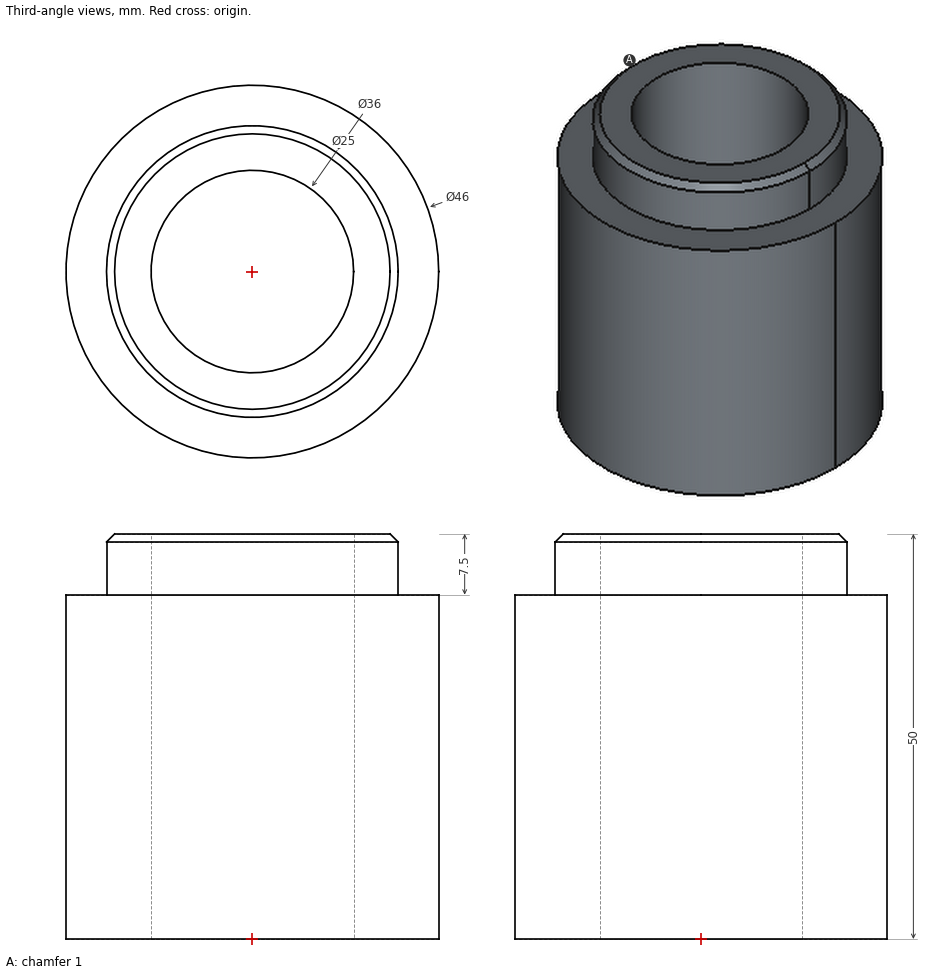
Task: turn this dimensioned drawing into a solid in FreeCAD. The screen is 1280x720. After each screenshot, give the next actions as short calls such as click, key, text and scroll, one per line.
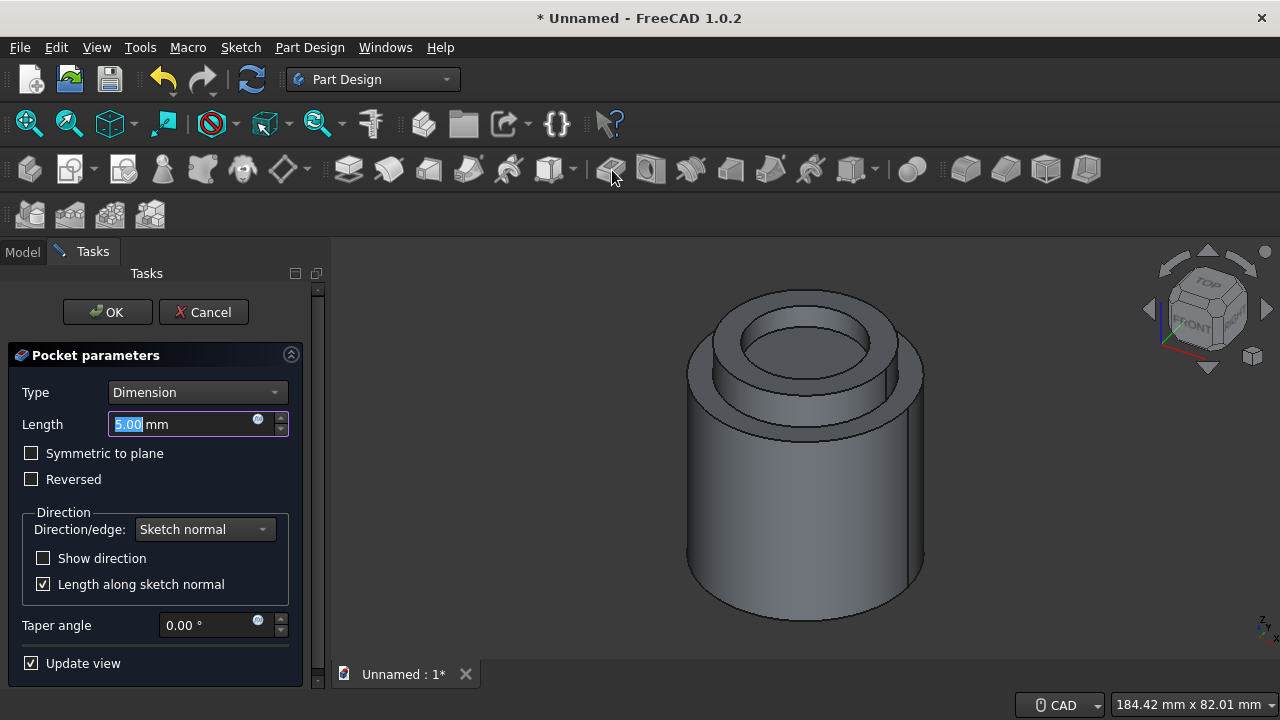
click(198, 392)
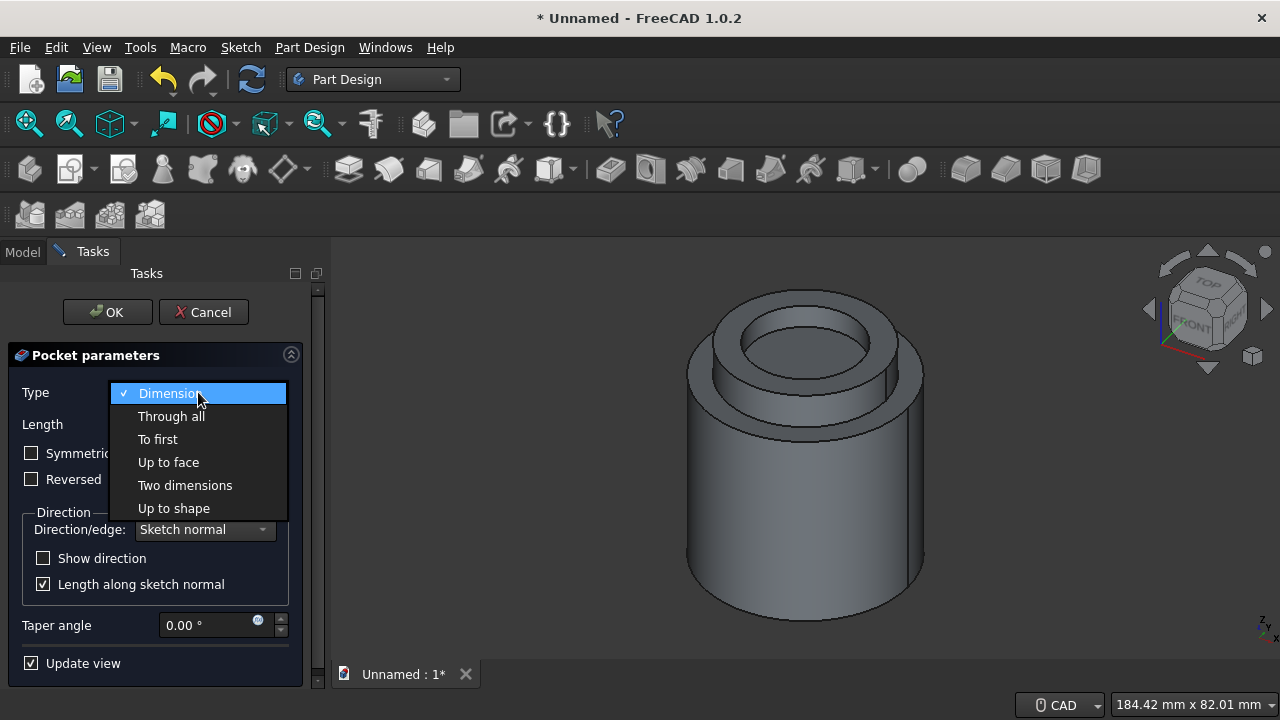
click(198, 416)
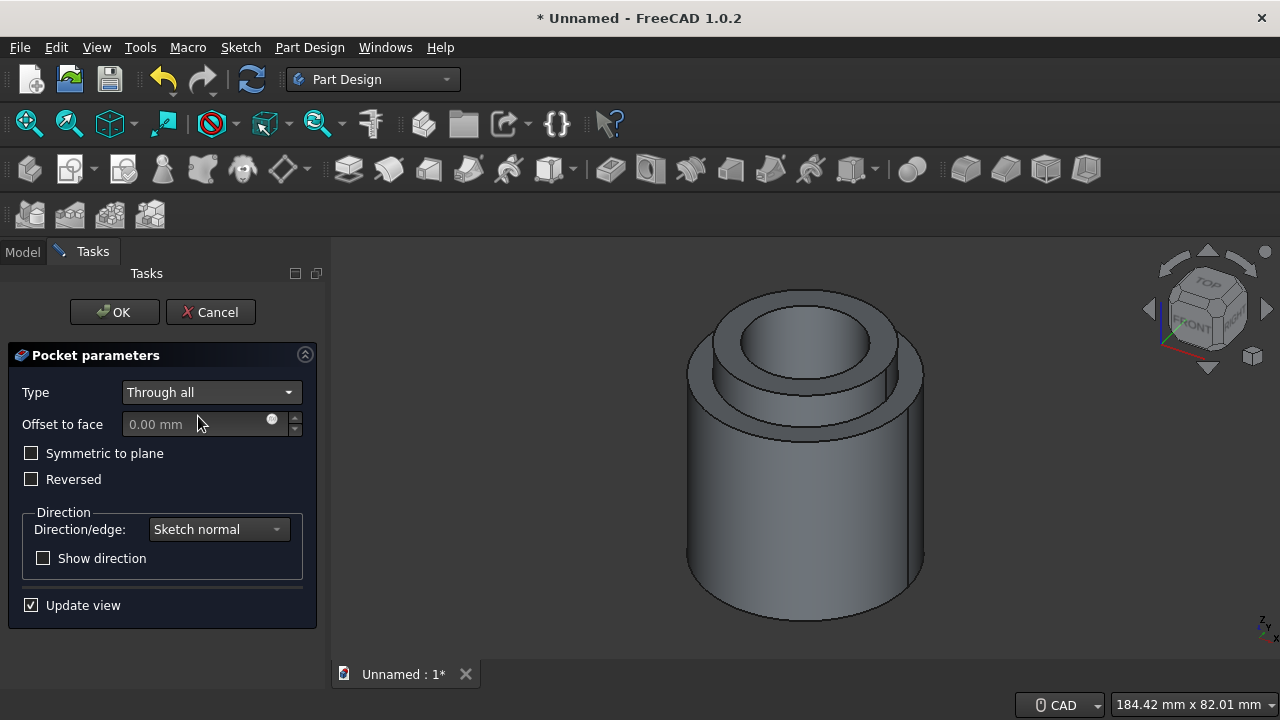
click(115, 312)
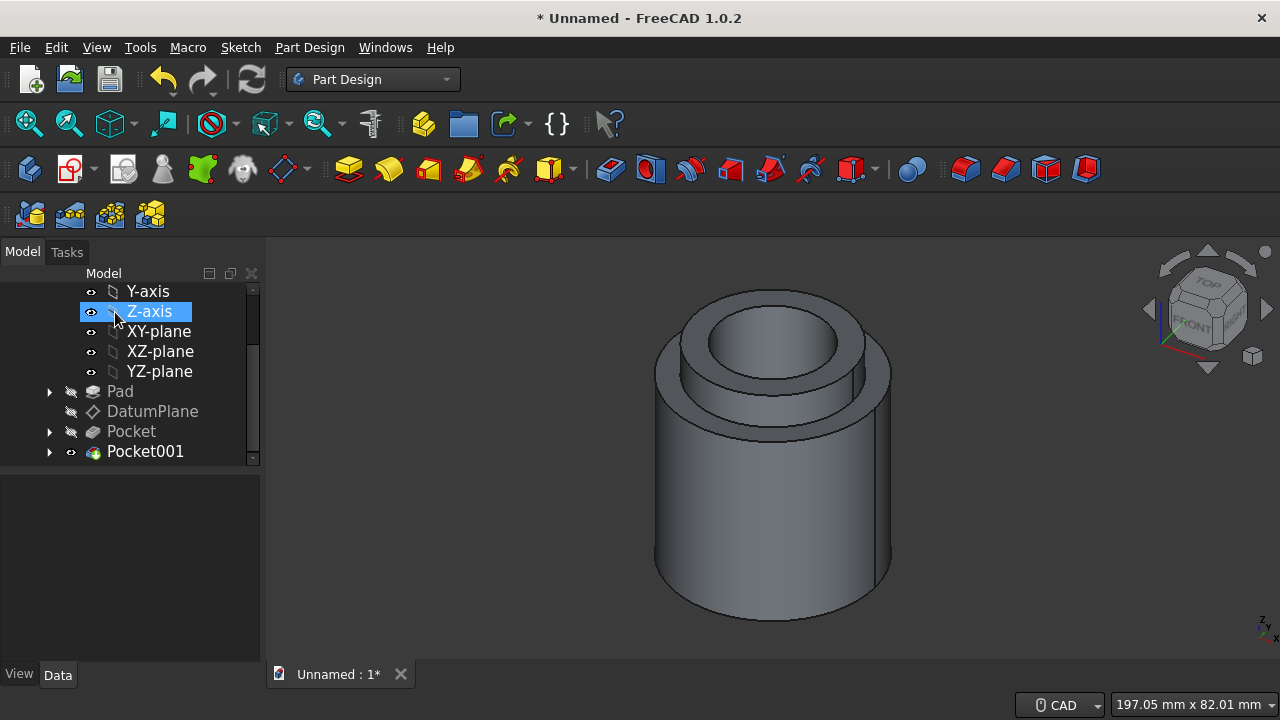
click(681, 347)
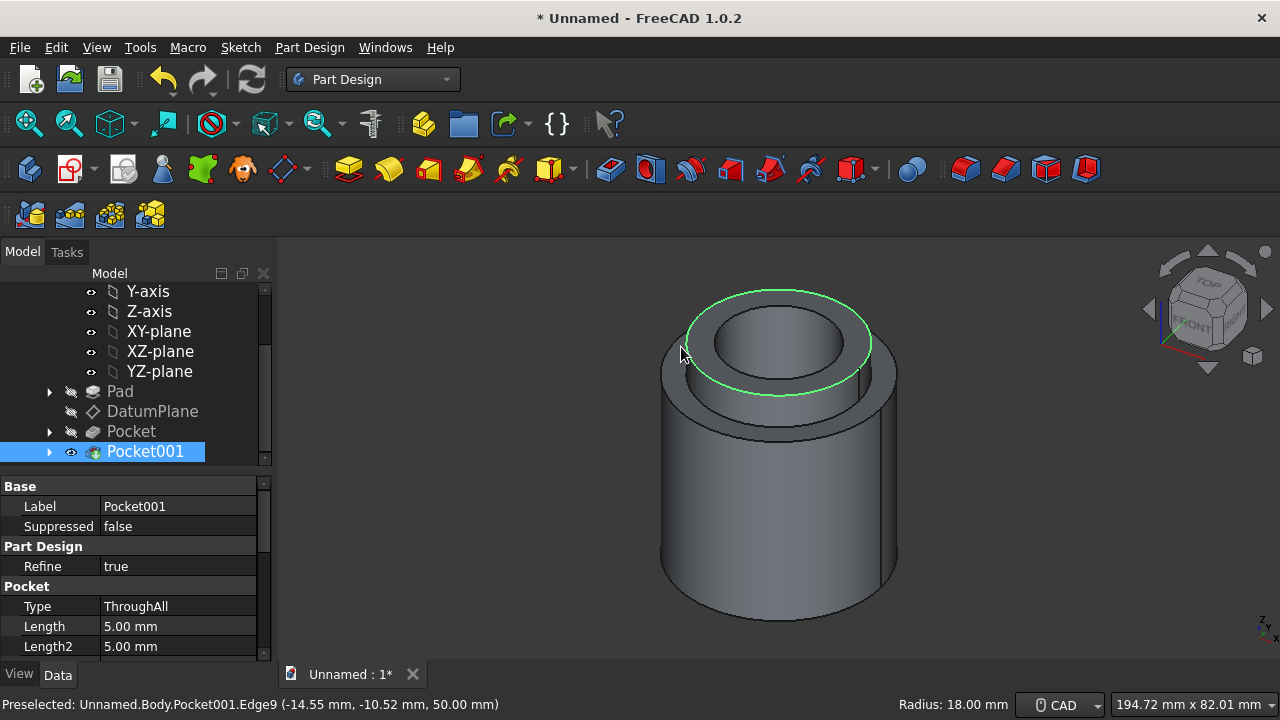
click(1006, 170)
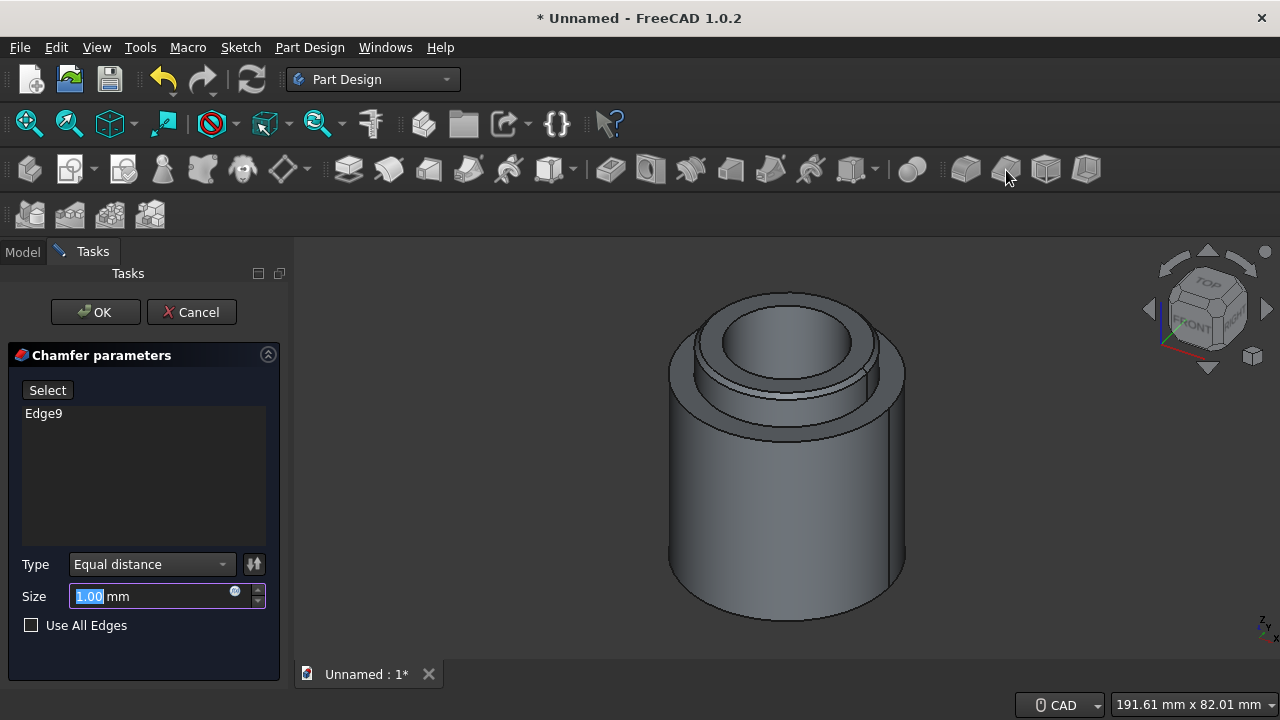
text(1)
key(Tab)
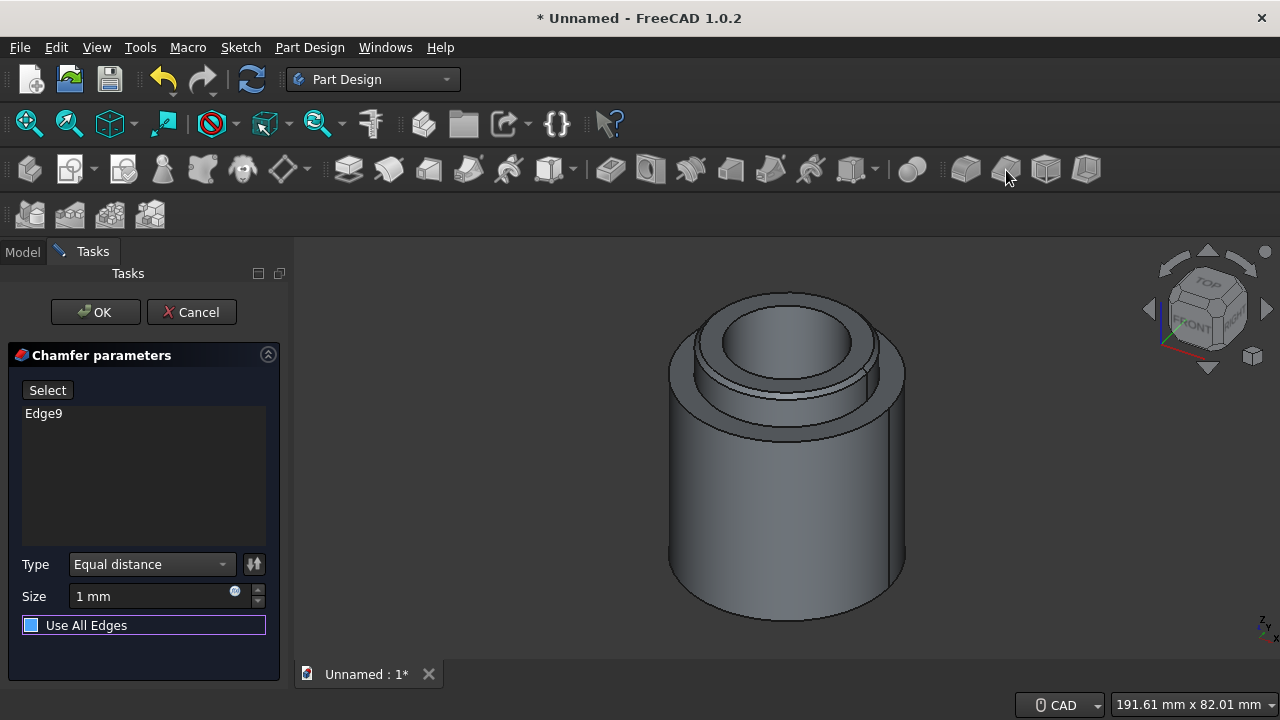
click(96, 312)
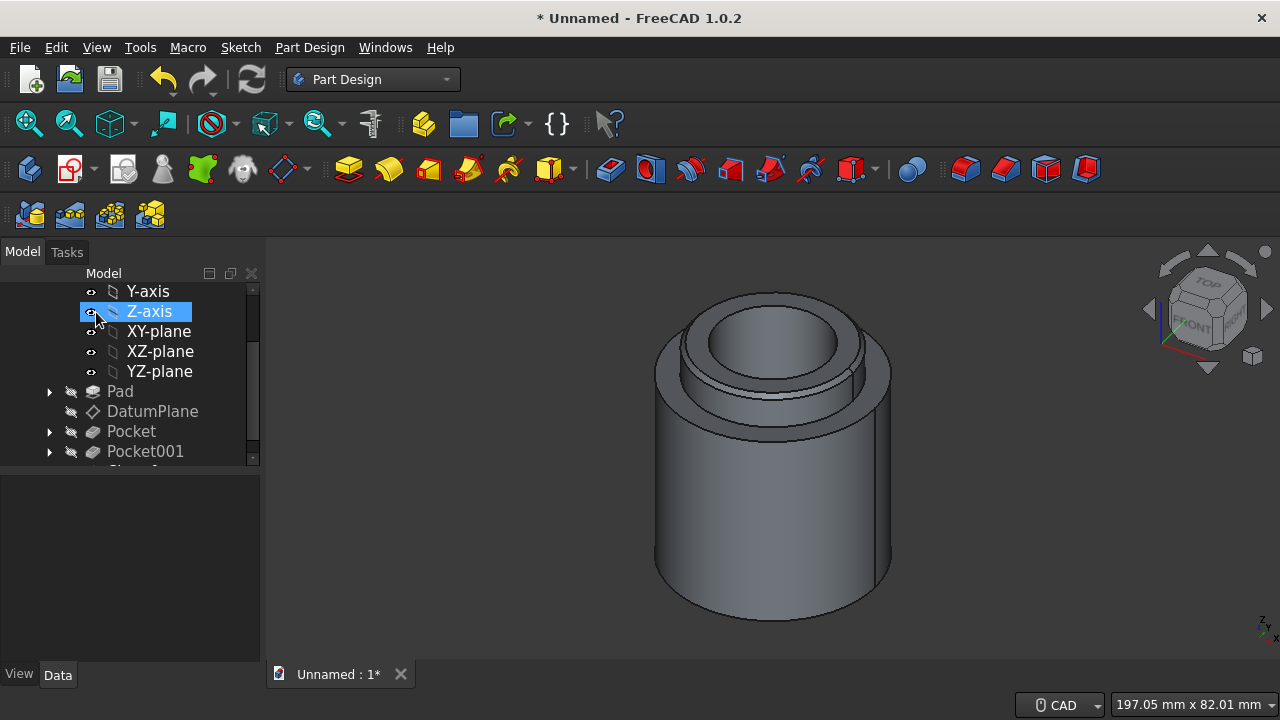
key(0)